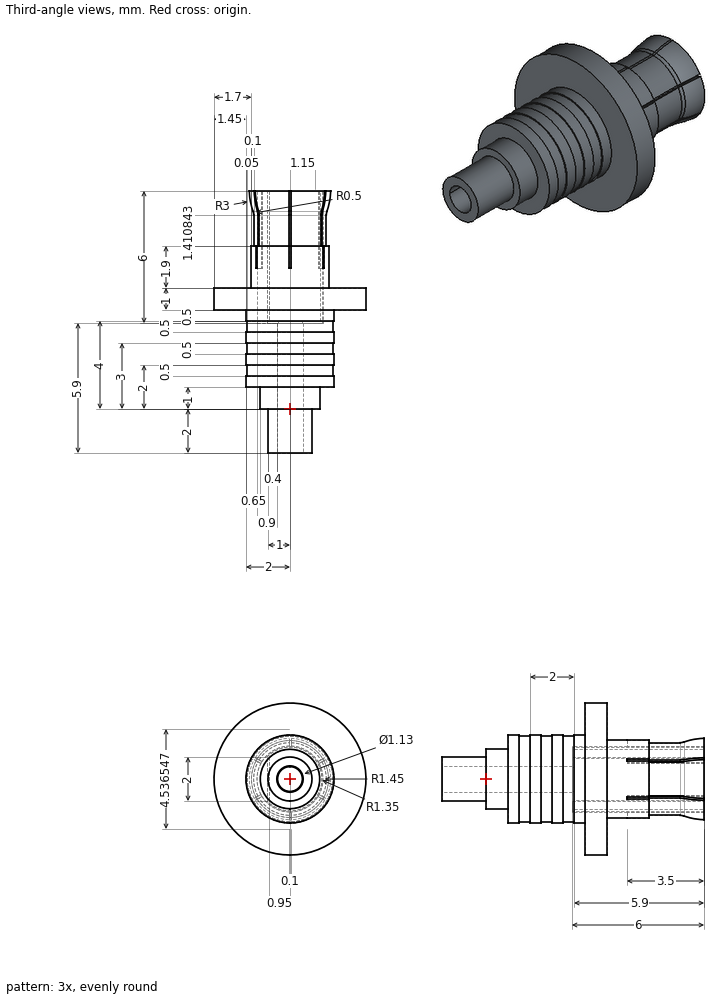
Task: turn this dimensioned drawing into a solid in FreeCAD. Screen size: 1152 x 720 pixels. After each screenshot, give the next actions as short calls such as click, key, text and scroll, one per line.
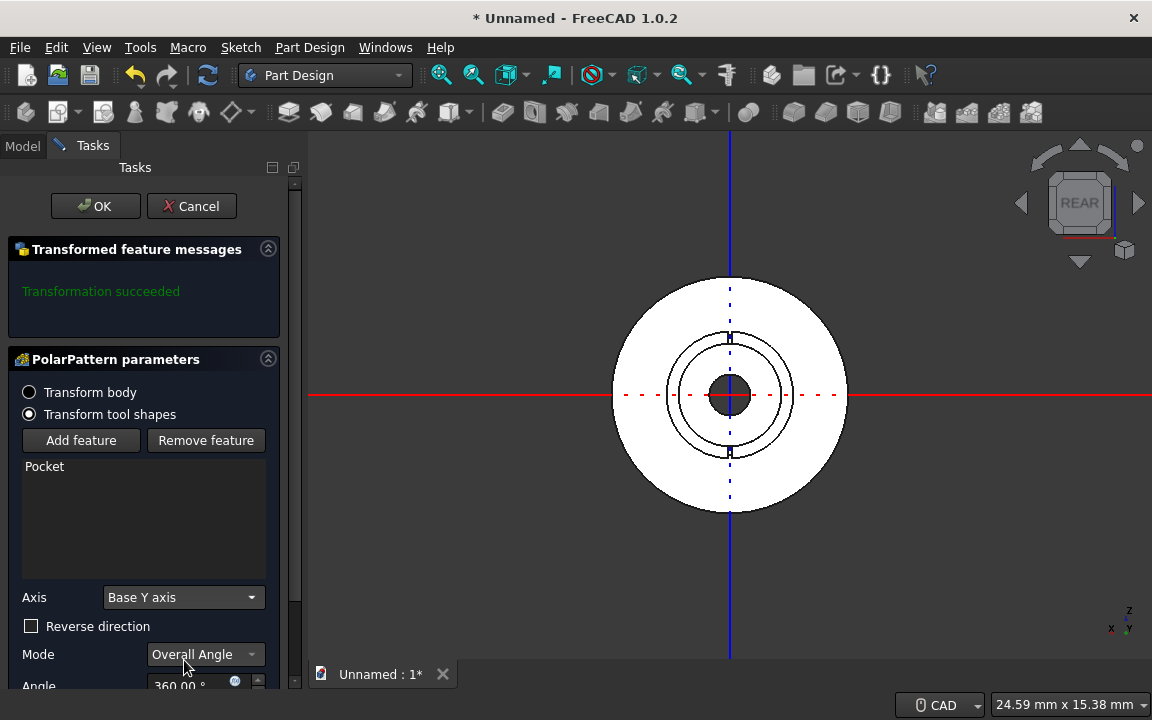
scroll(295, 432, down, 2)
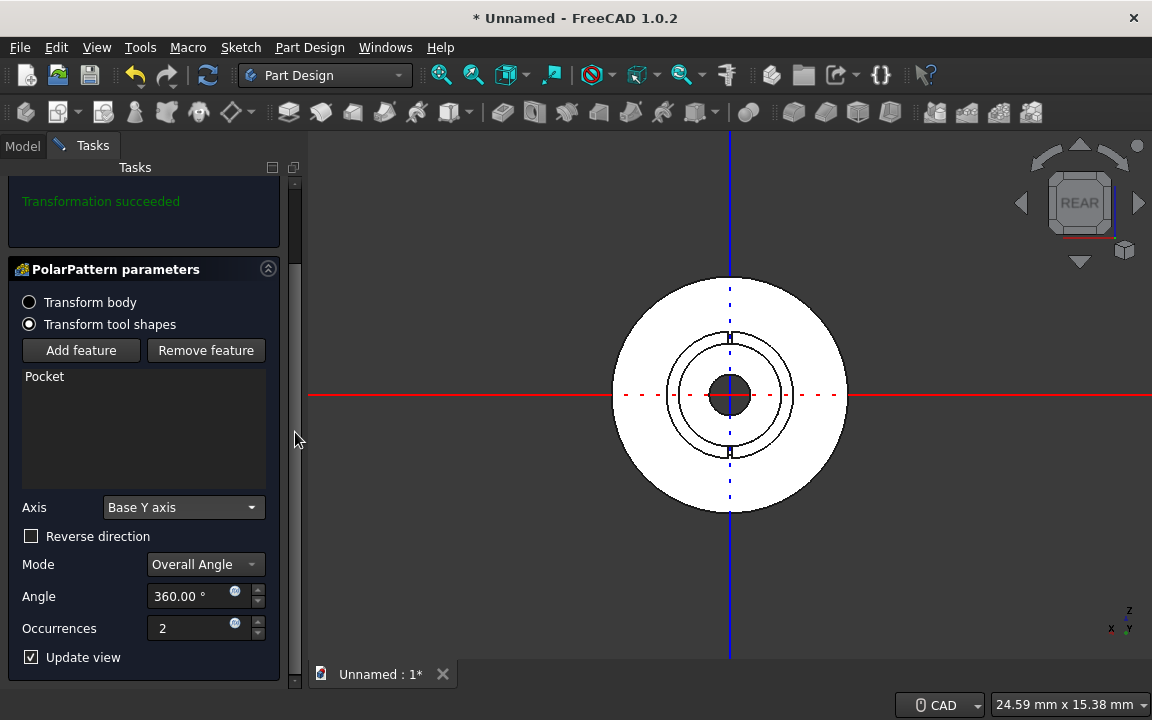
triple_click(198, 628)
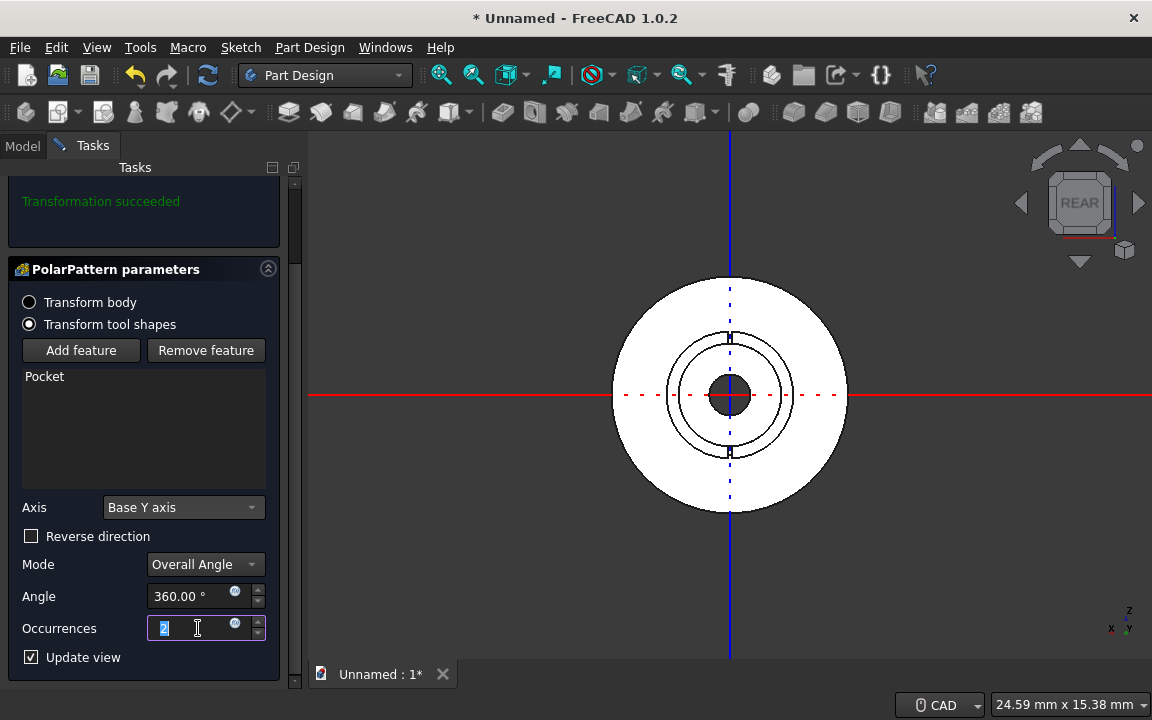
text(3)
key(Tab)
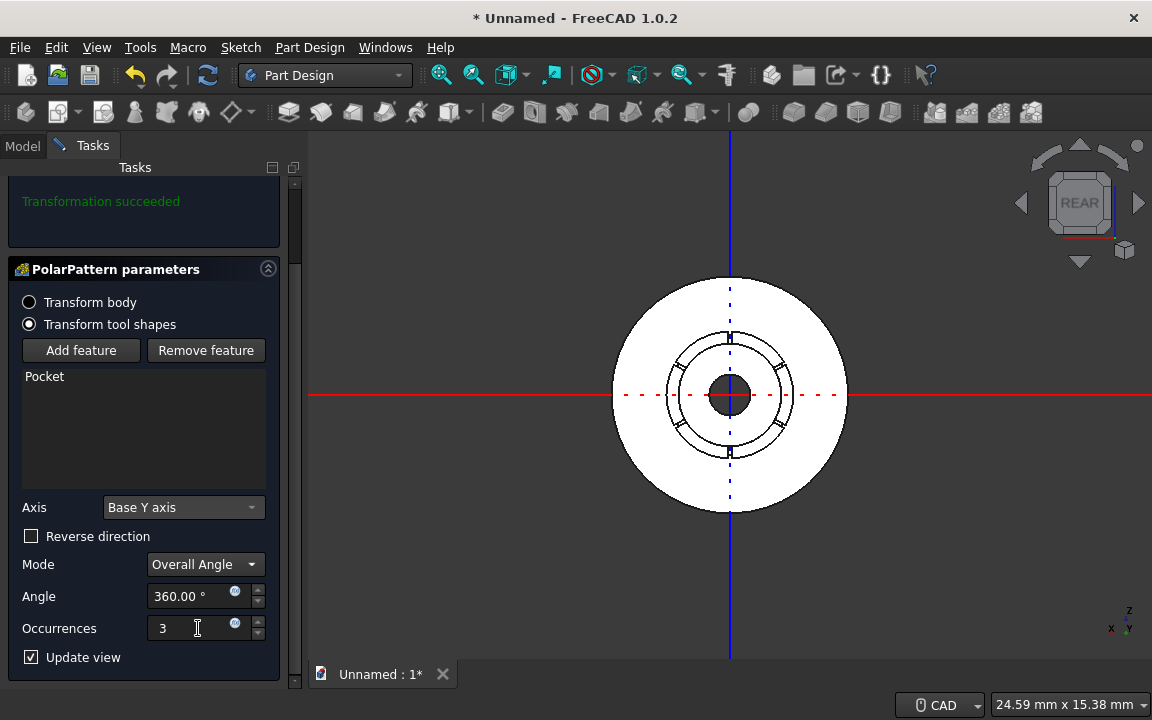
scroll(295, 432, up, 3)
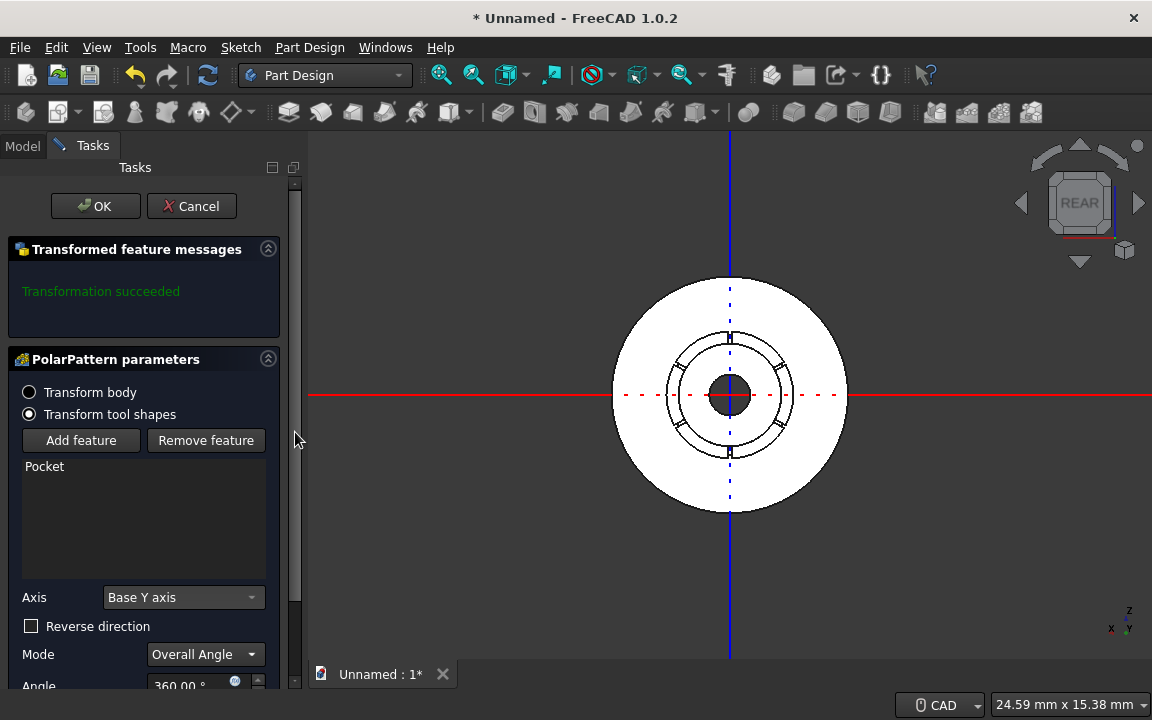
click(96, 206)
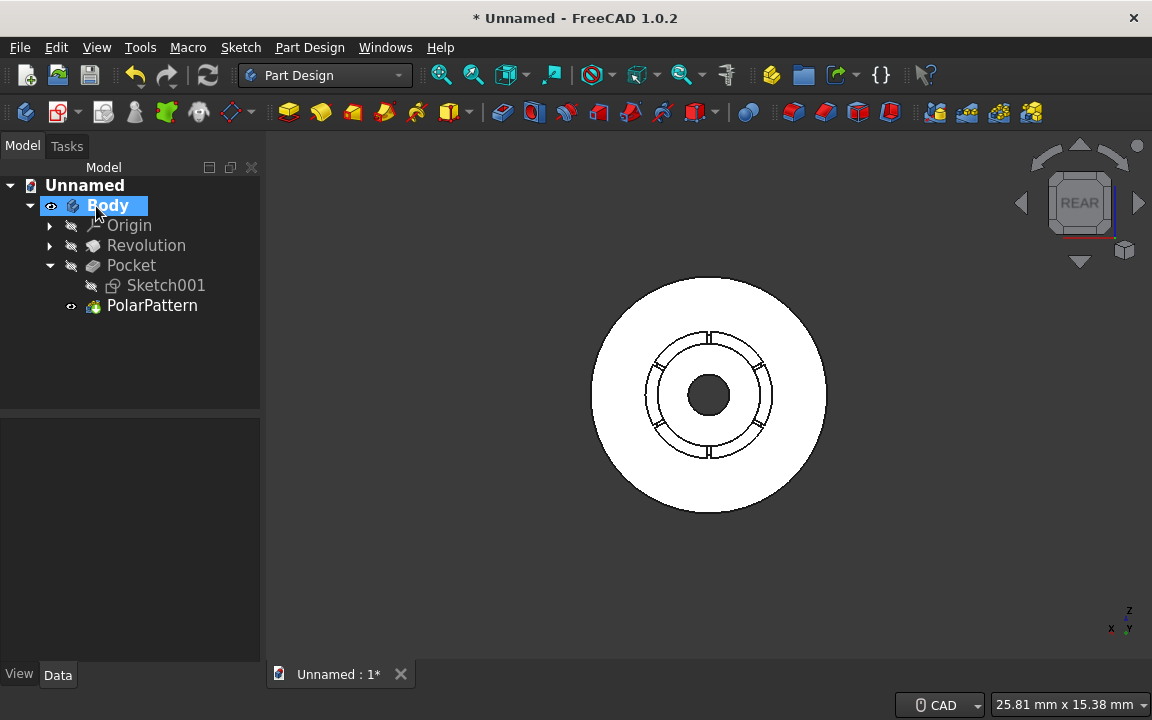
click(442, 76)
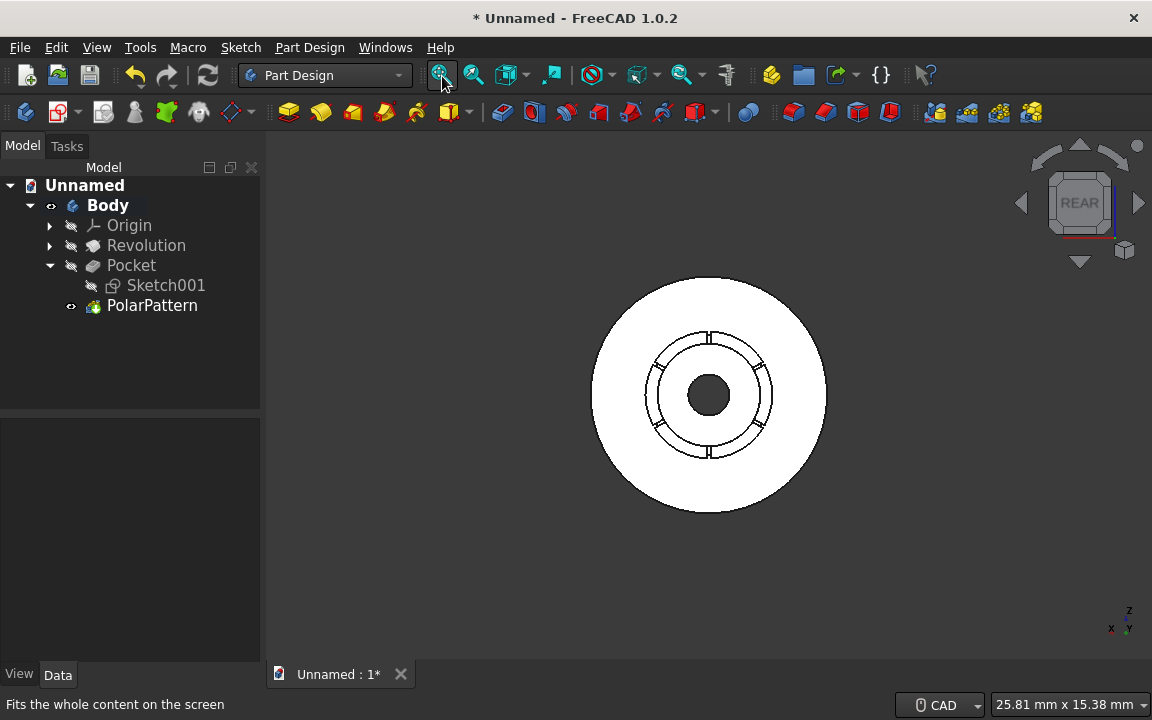
click(694, 365)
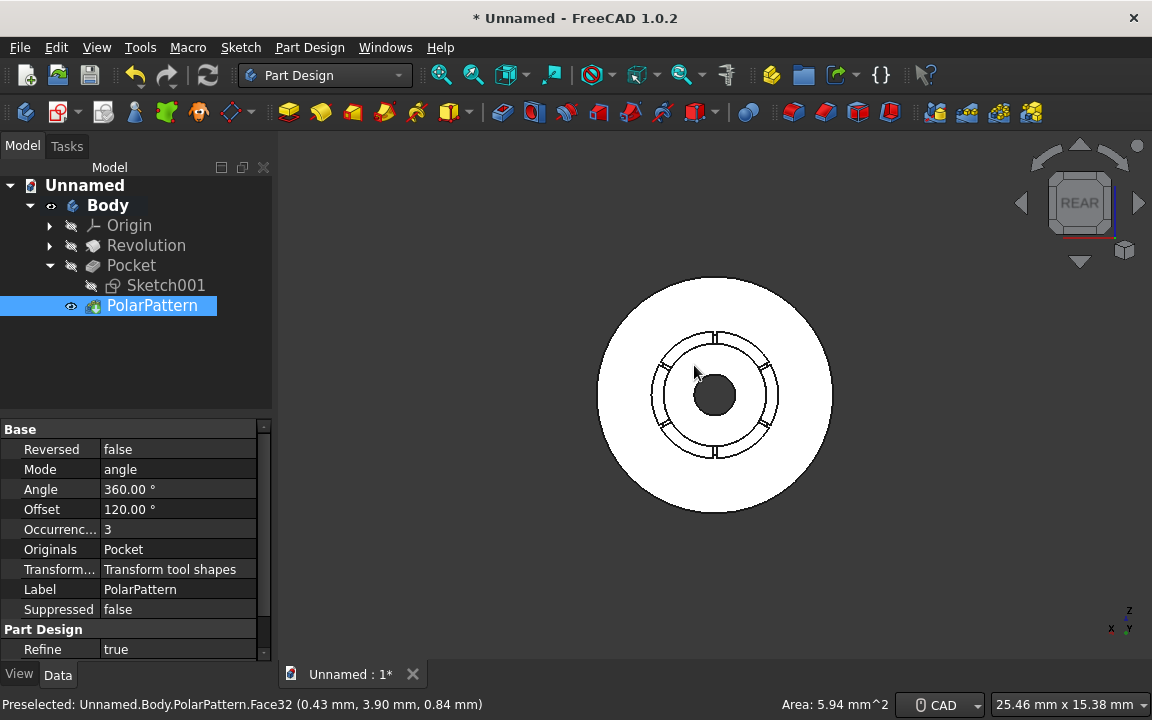
click(58, 112)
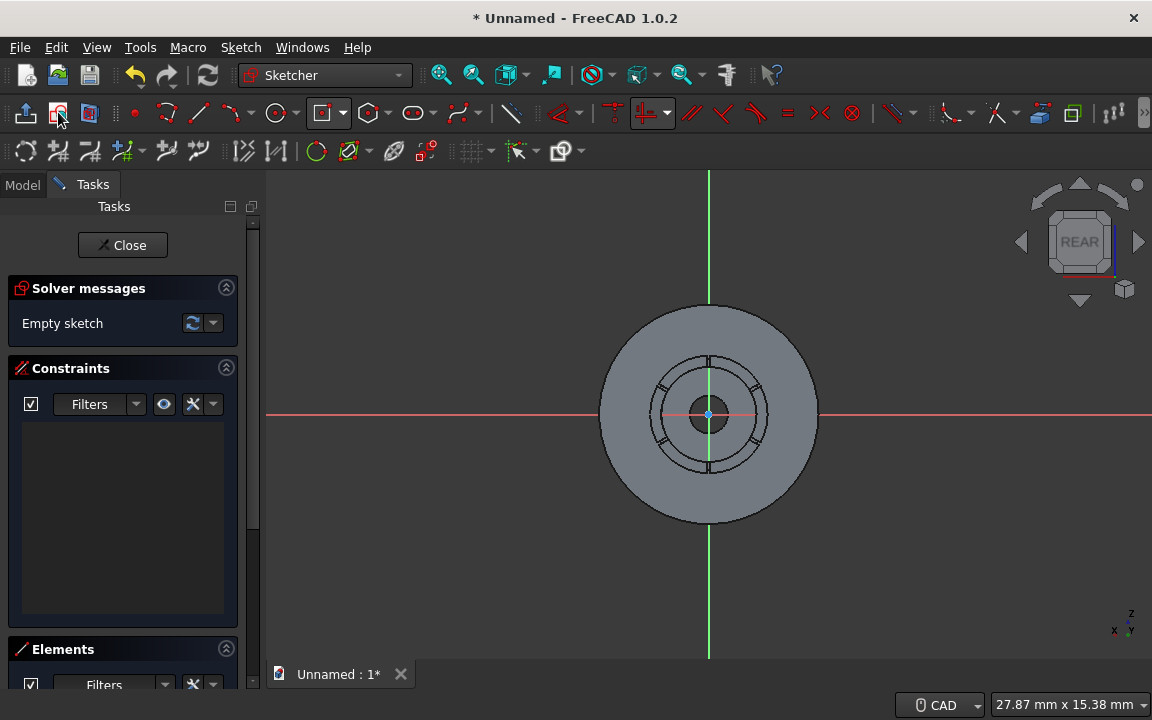
scroll(718, 414, up, 8)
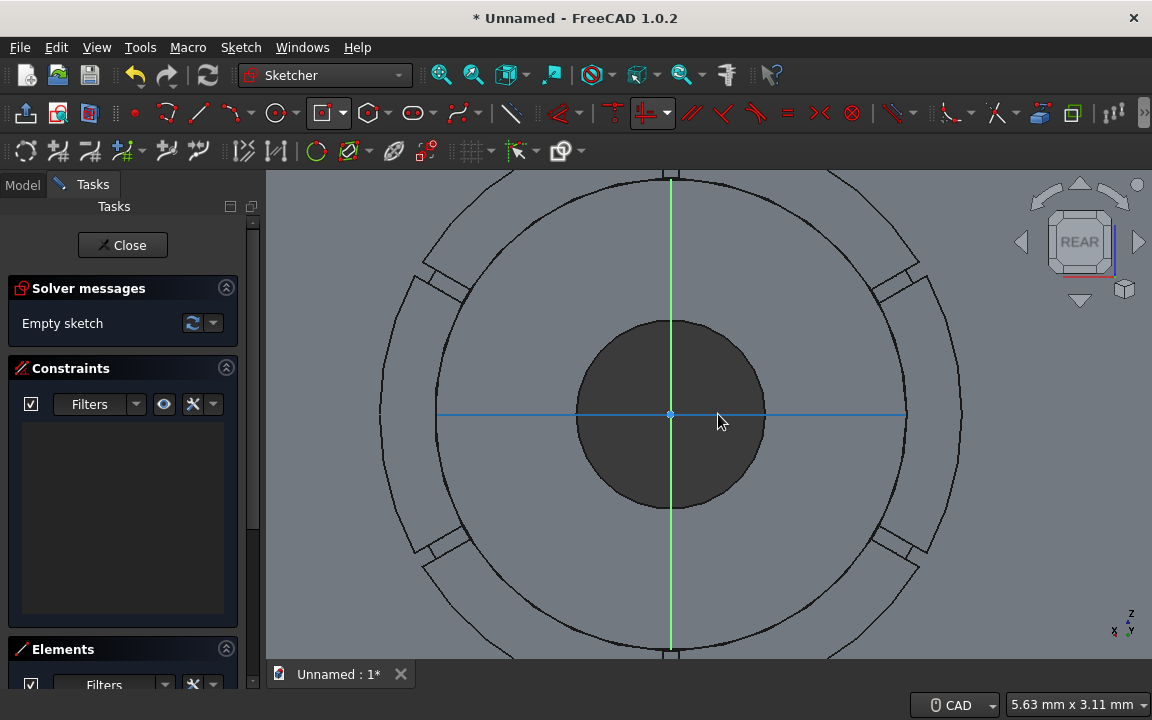
click(200, 114)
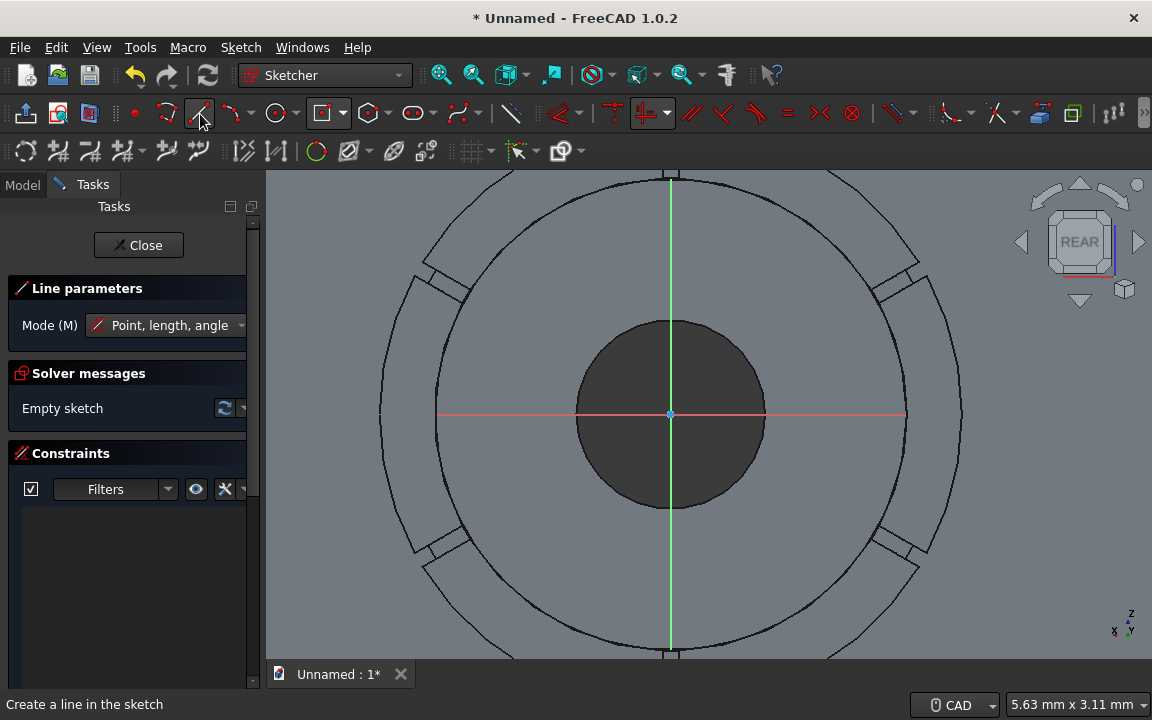
click(836, 572)
click(836, 257)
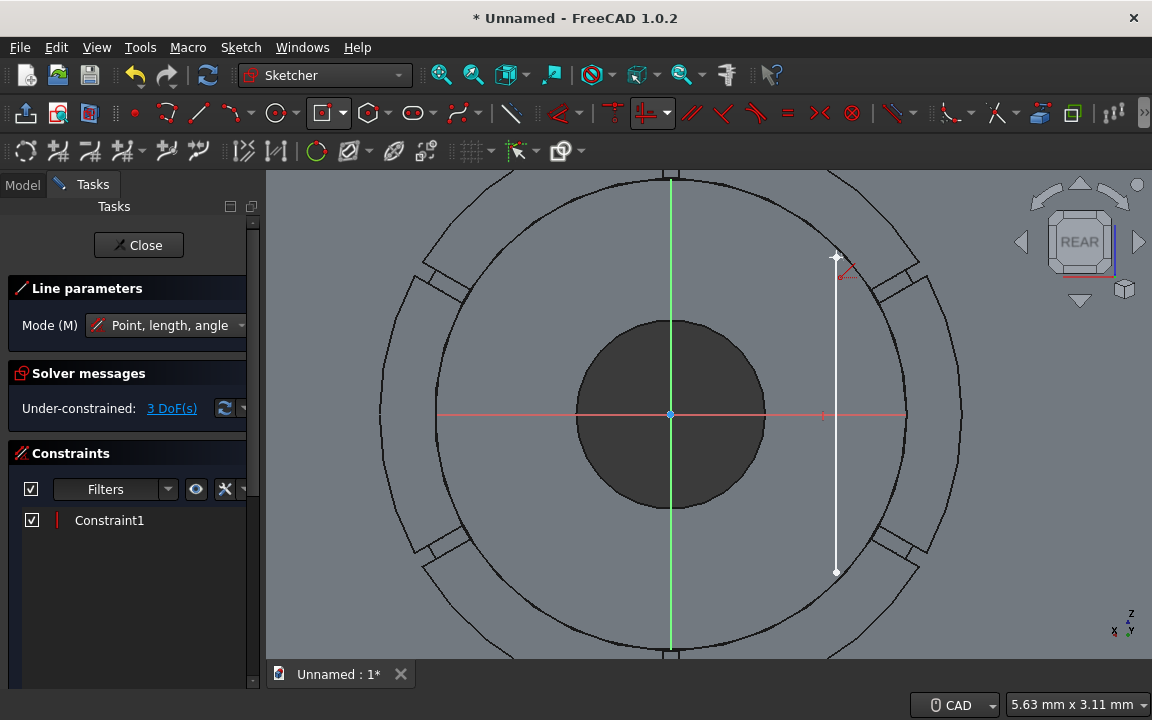
click(232, 114)